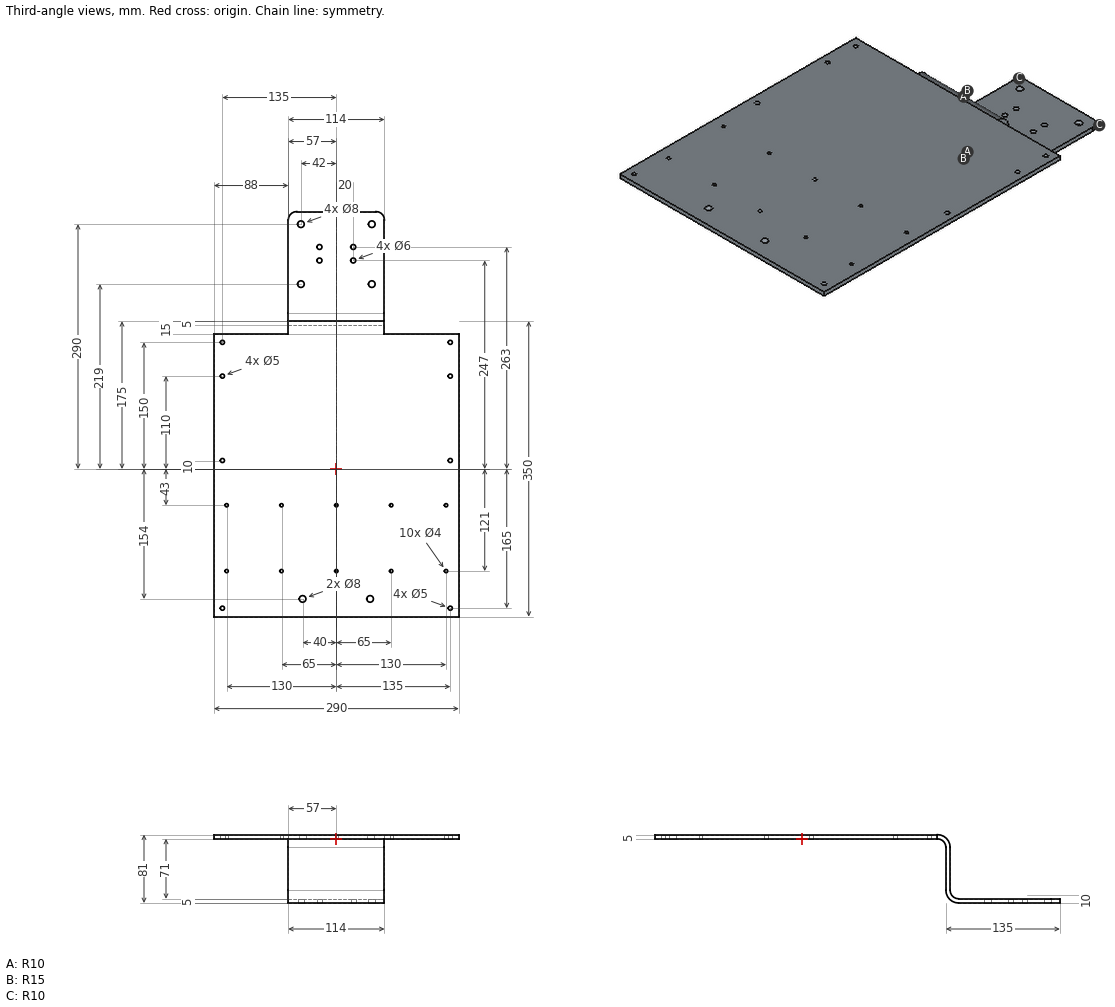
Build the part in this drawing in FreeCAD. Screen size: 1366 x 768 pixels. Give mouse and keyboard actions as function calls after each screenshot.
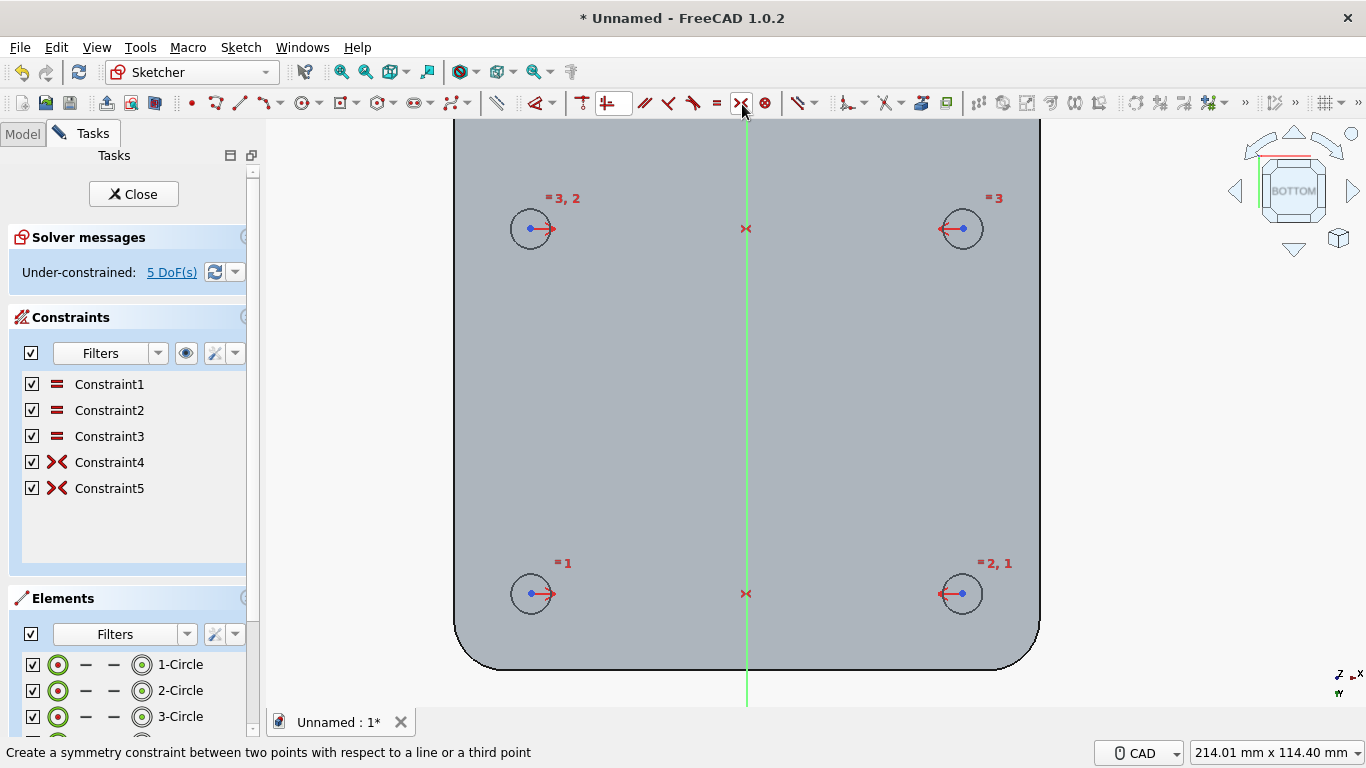
key(d)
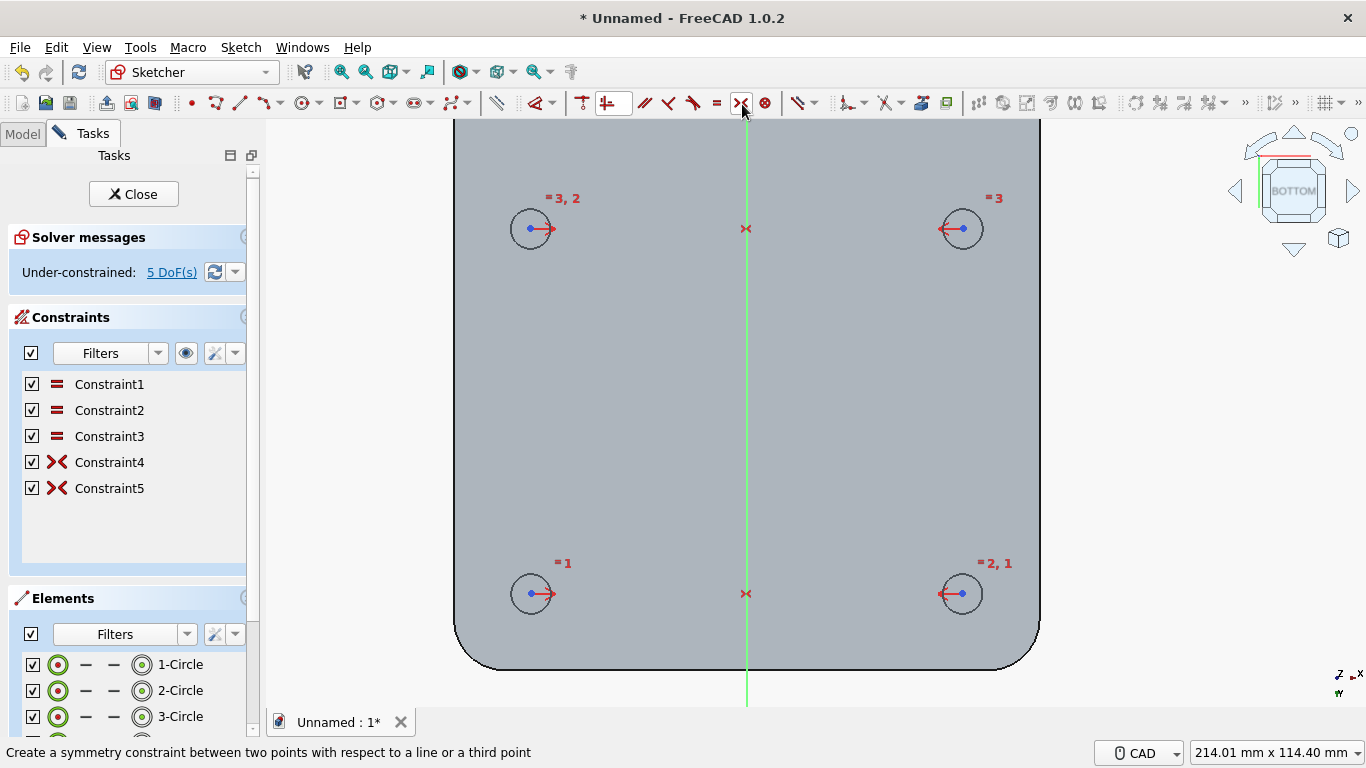
click(545, 580)
click(568, 557)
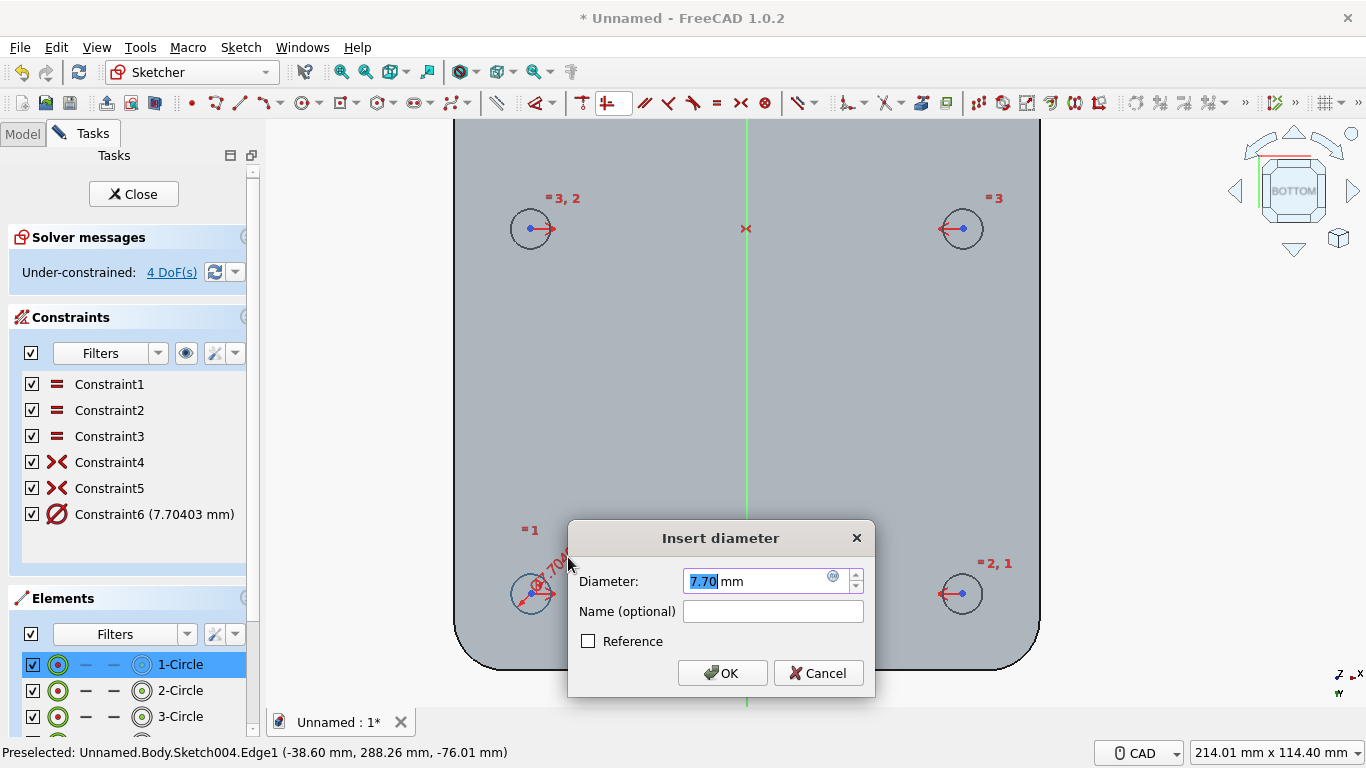
text(8)
key(Return)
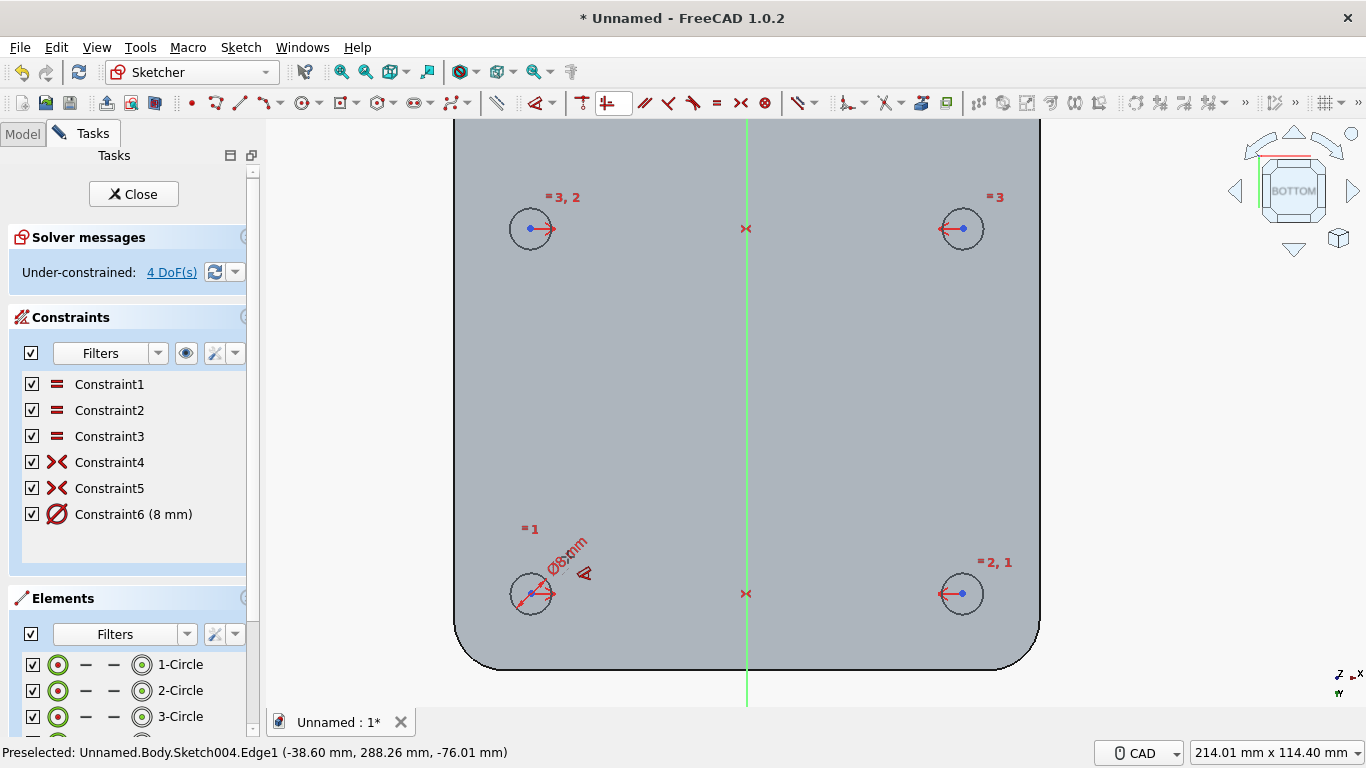
click(531, 594)
click(639, 628)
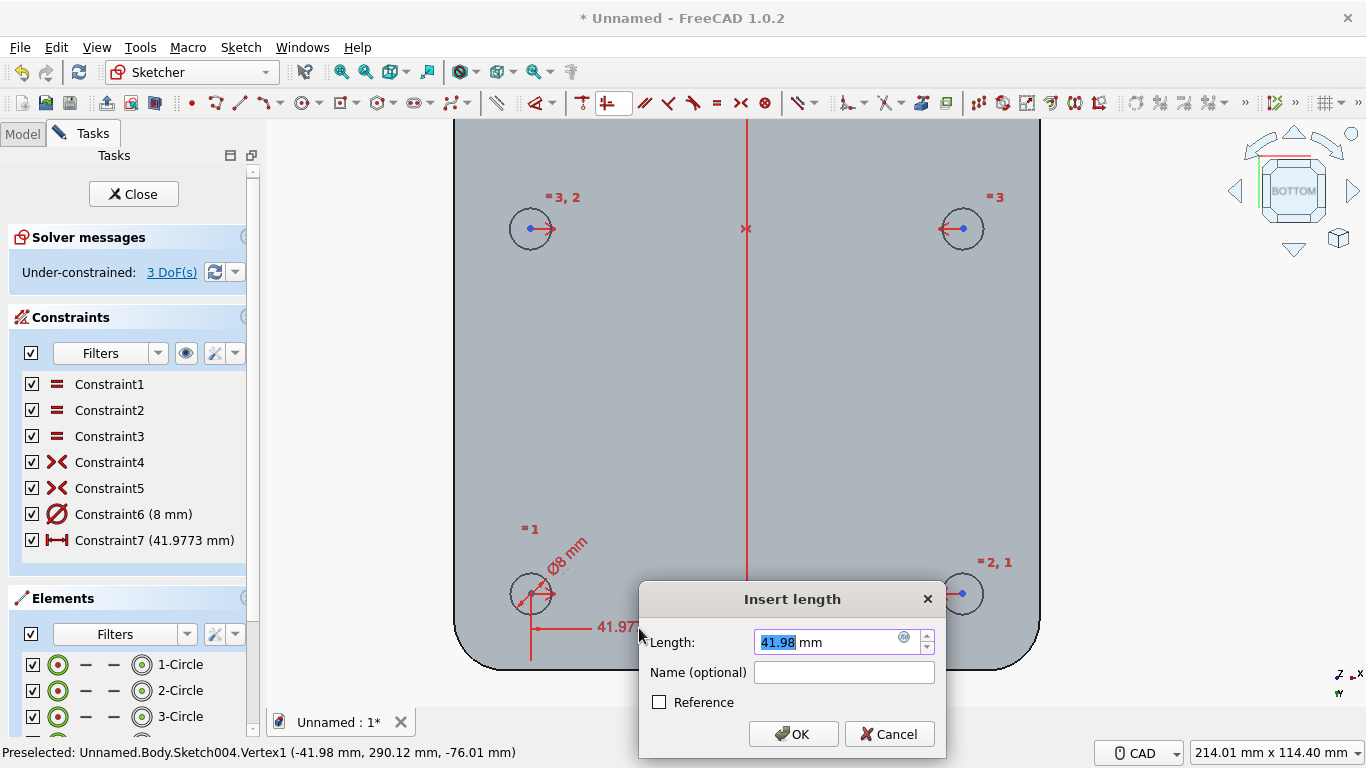
text(42)
key(Return)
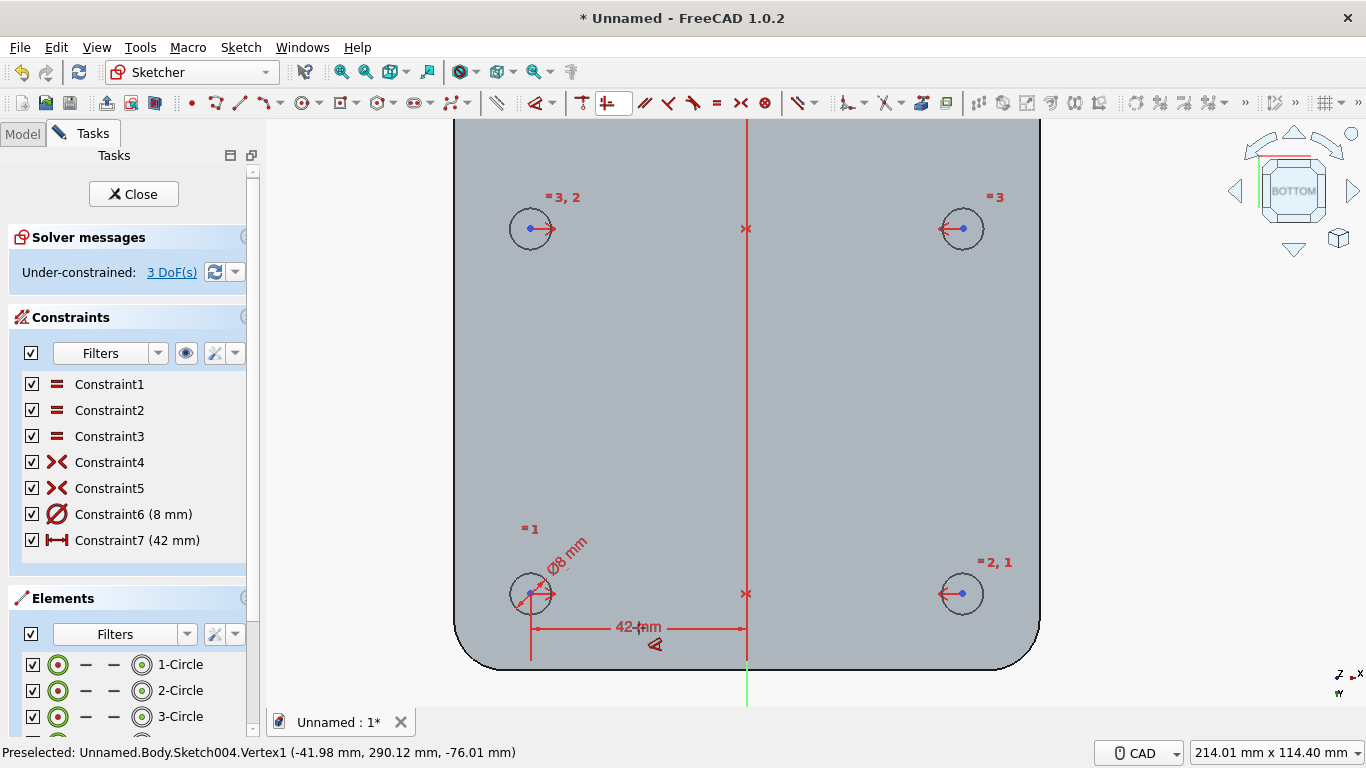
click(531, 229)
click(639, 263)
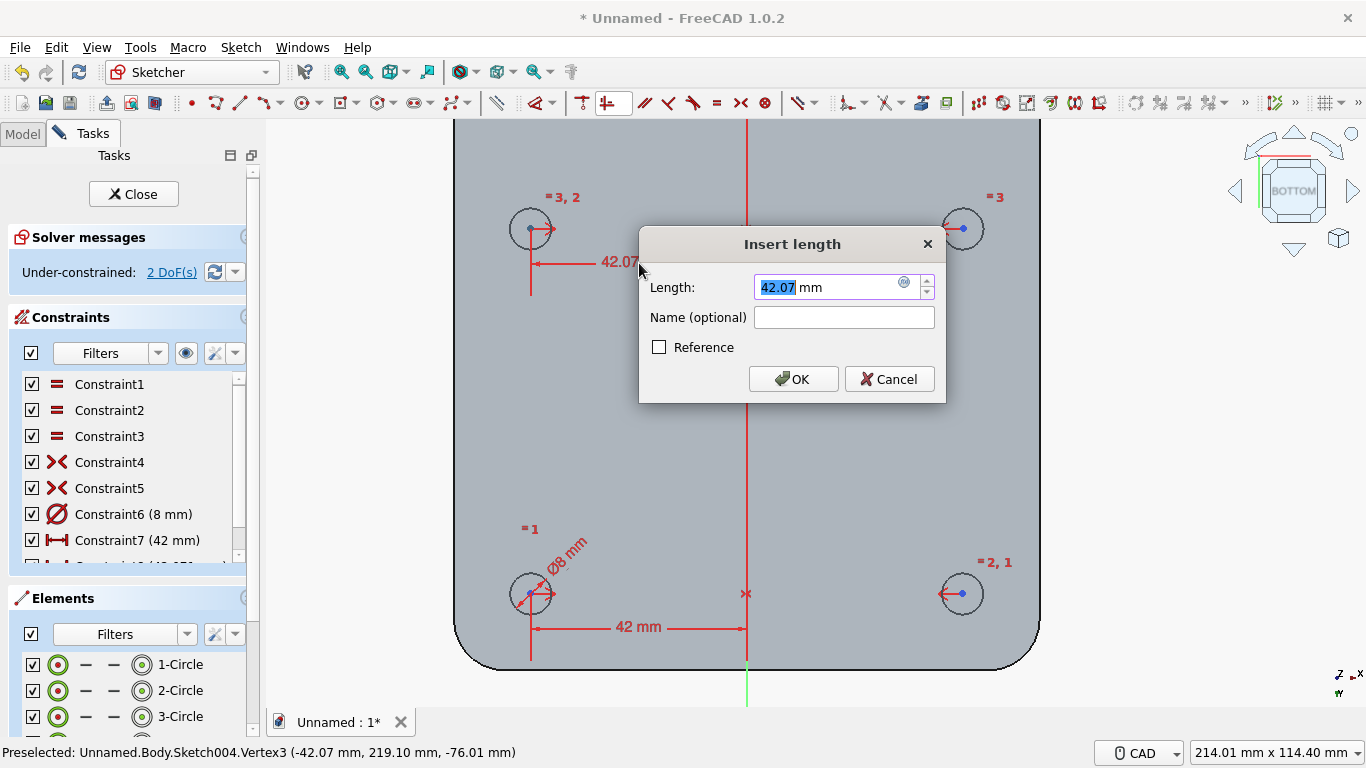
text(42)
key(Return)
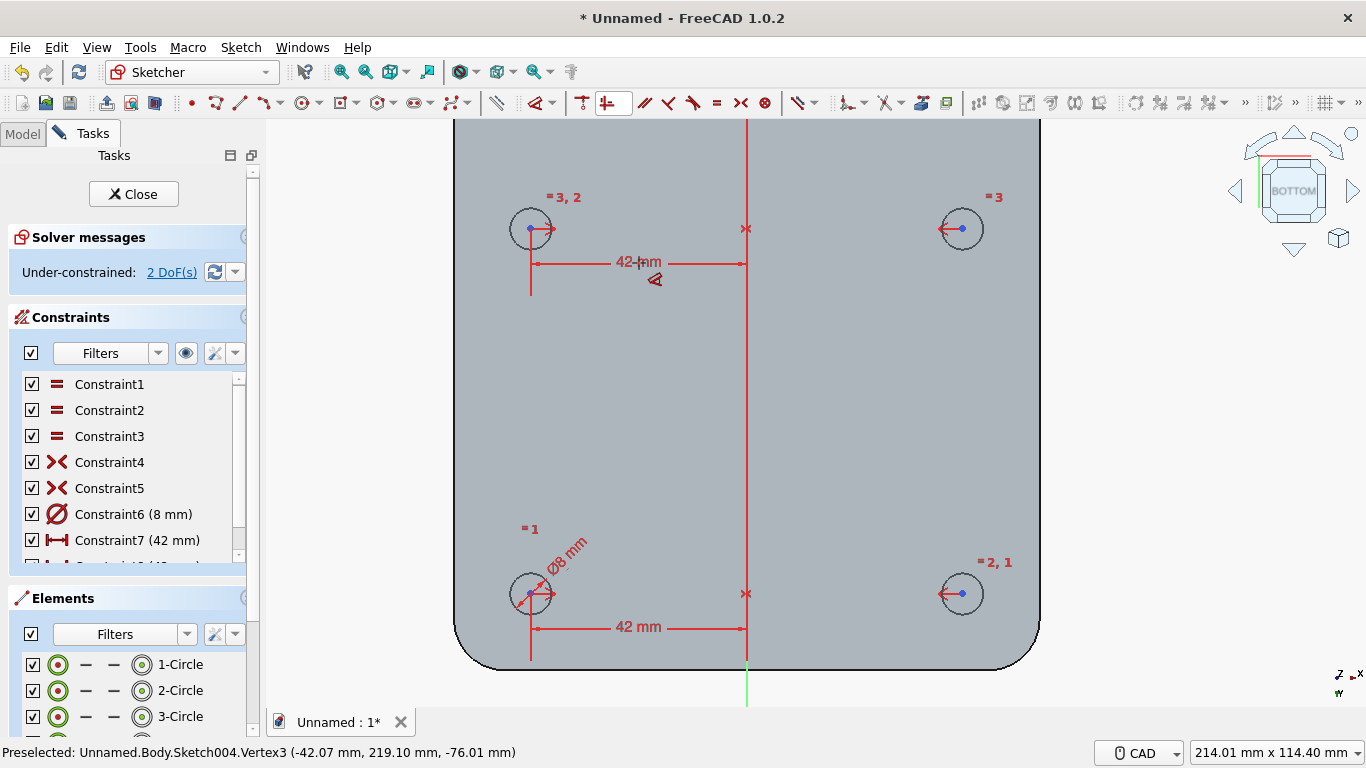
click(531, 594)
click(497, 370)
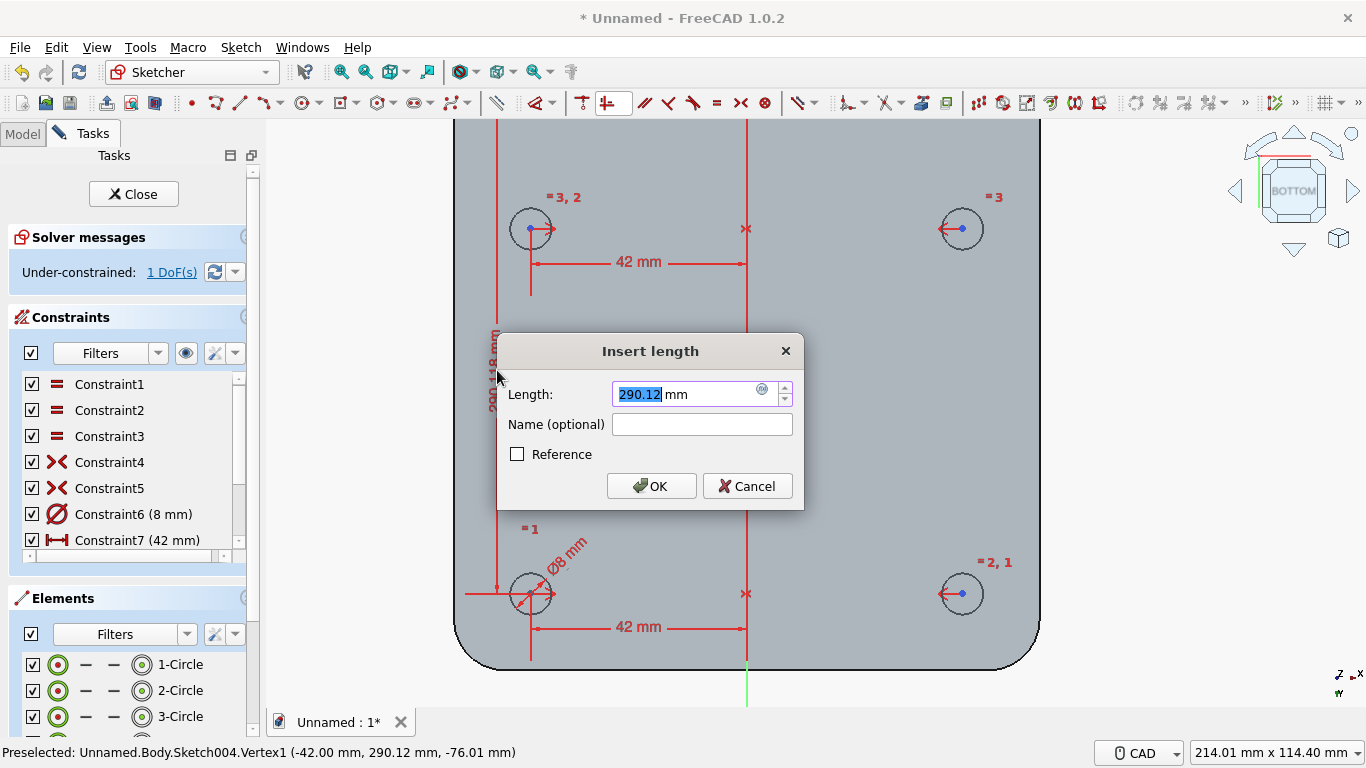
text(290)
key(Return)